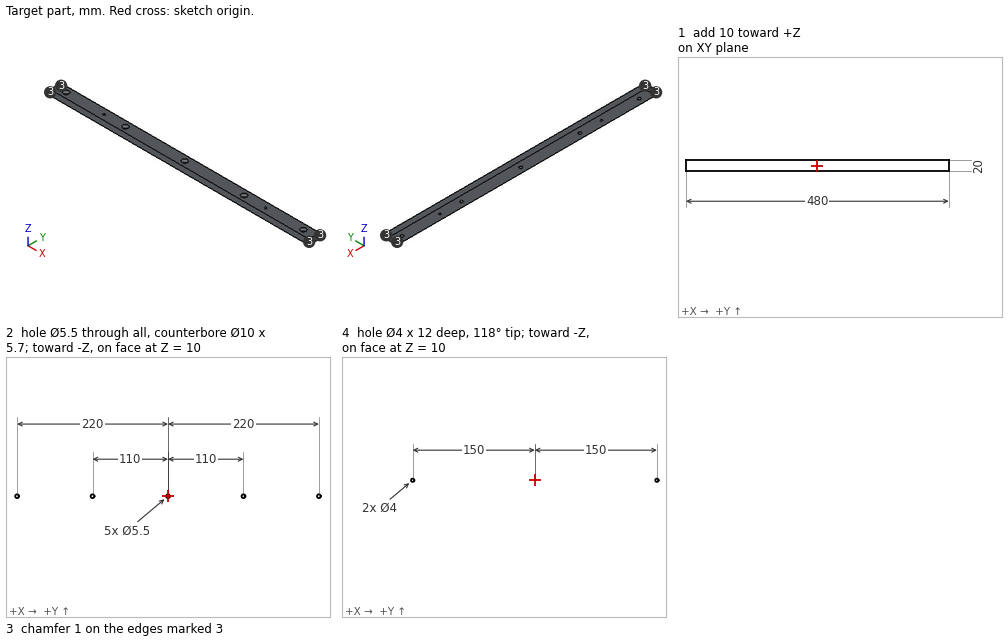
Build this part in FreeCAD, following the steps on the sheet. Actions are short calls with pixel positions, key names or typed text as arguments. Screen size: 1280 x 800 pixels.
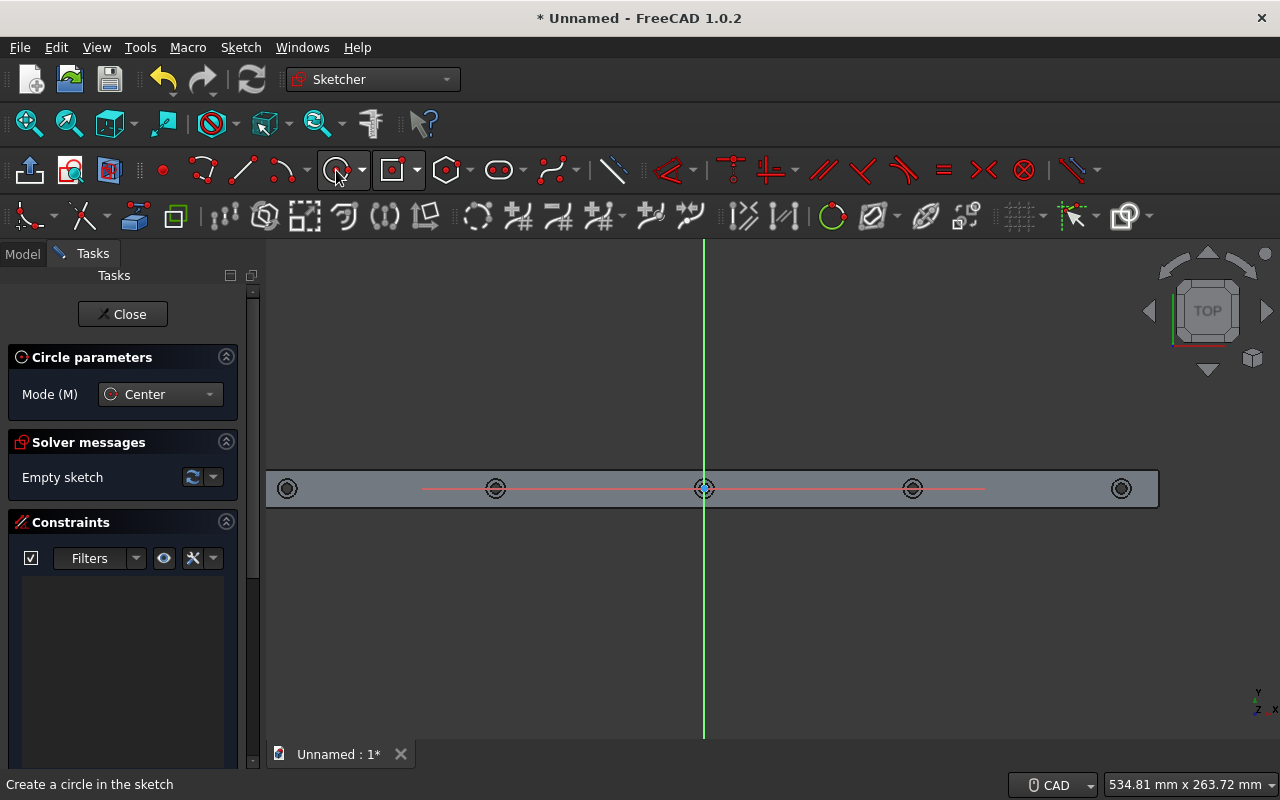
scroll(420, 489, up, 9)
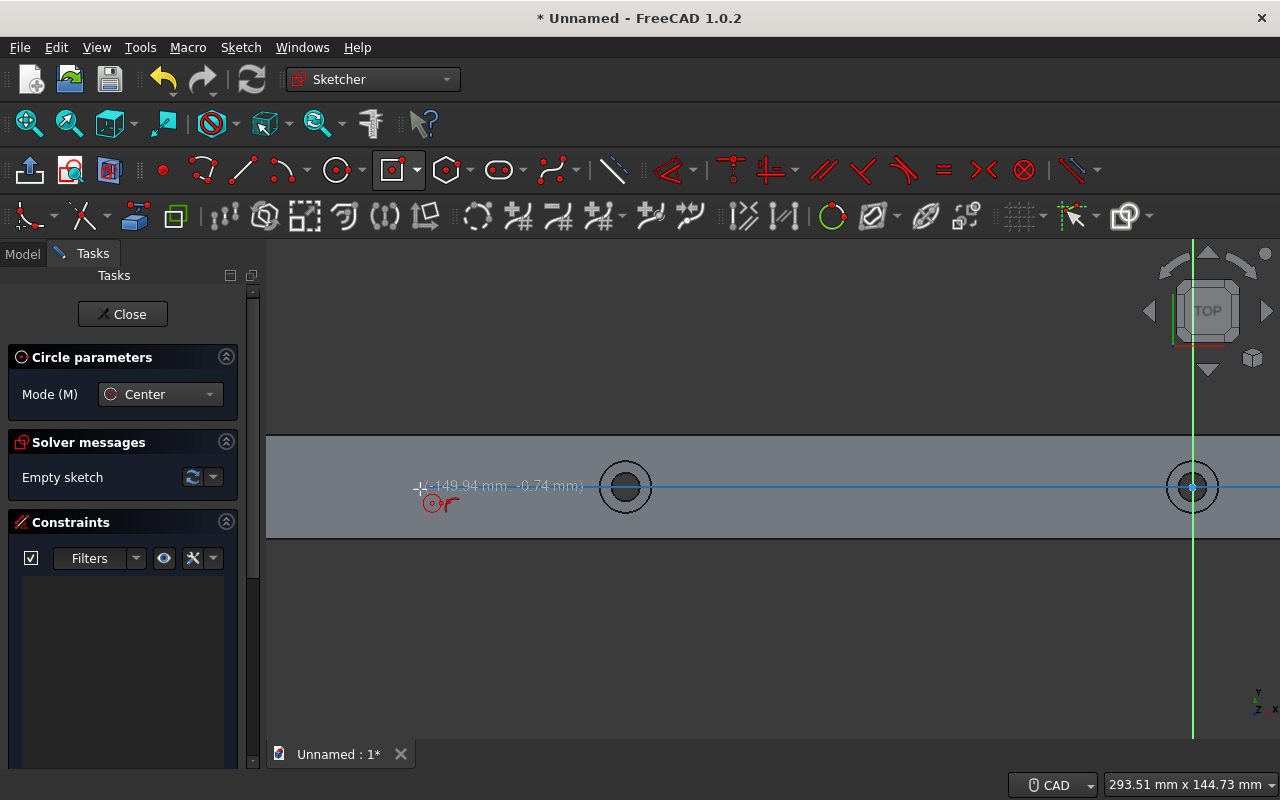
scroll(420, 490, down, 9)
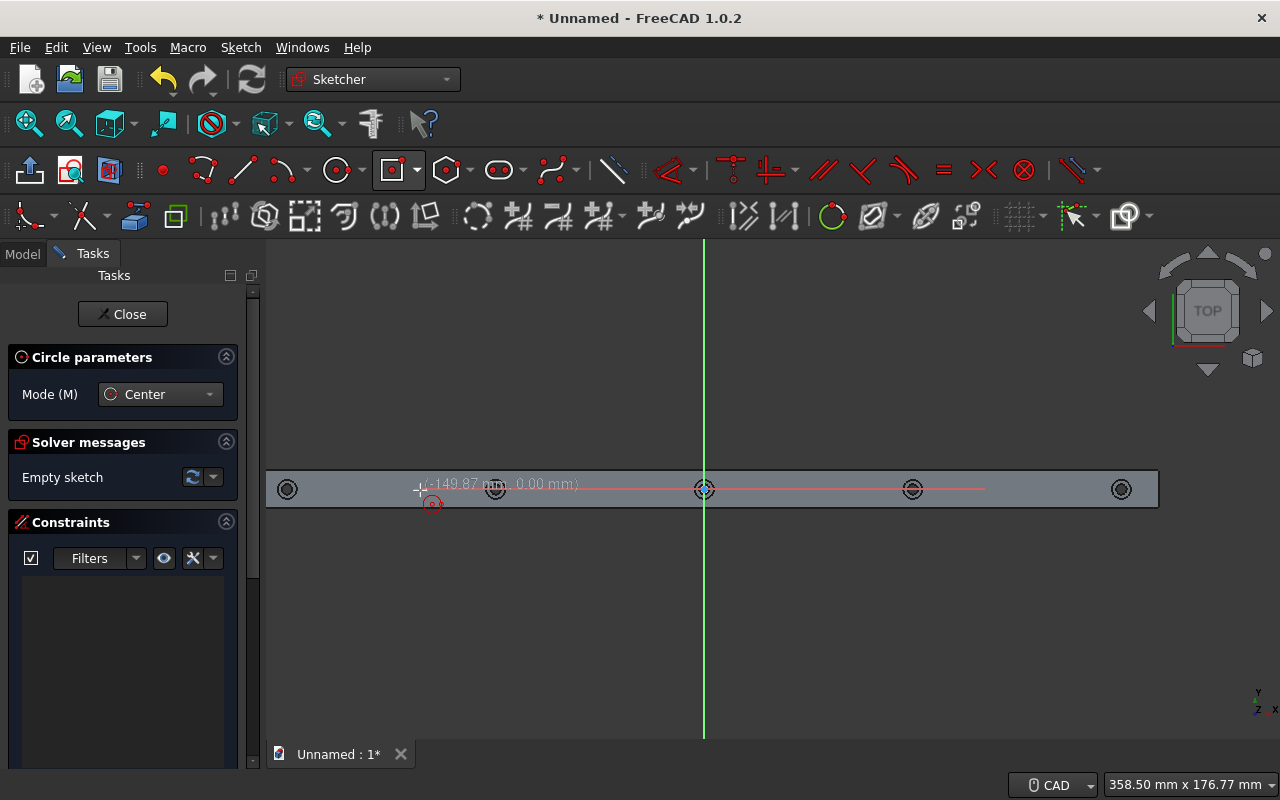
click(420, 489)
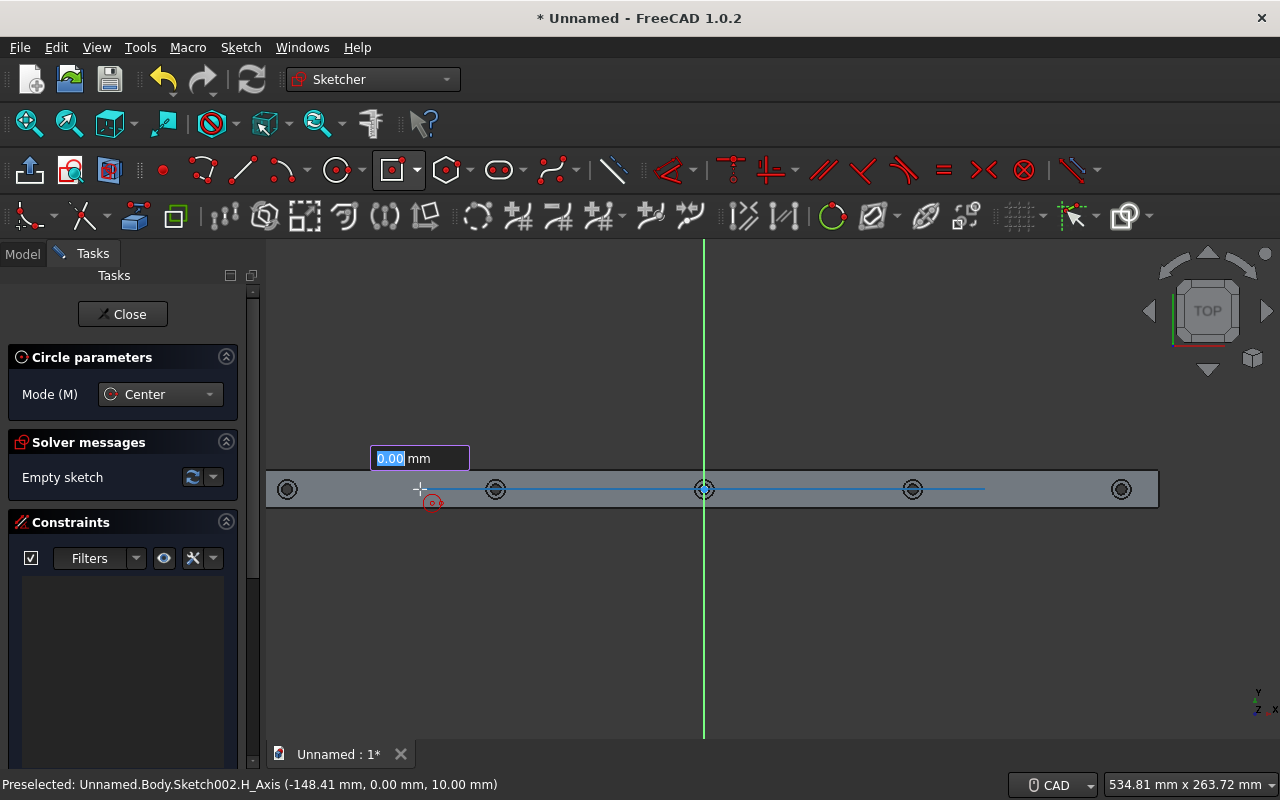
scroll(419, 493, up, 8)
move(416, 491)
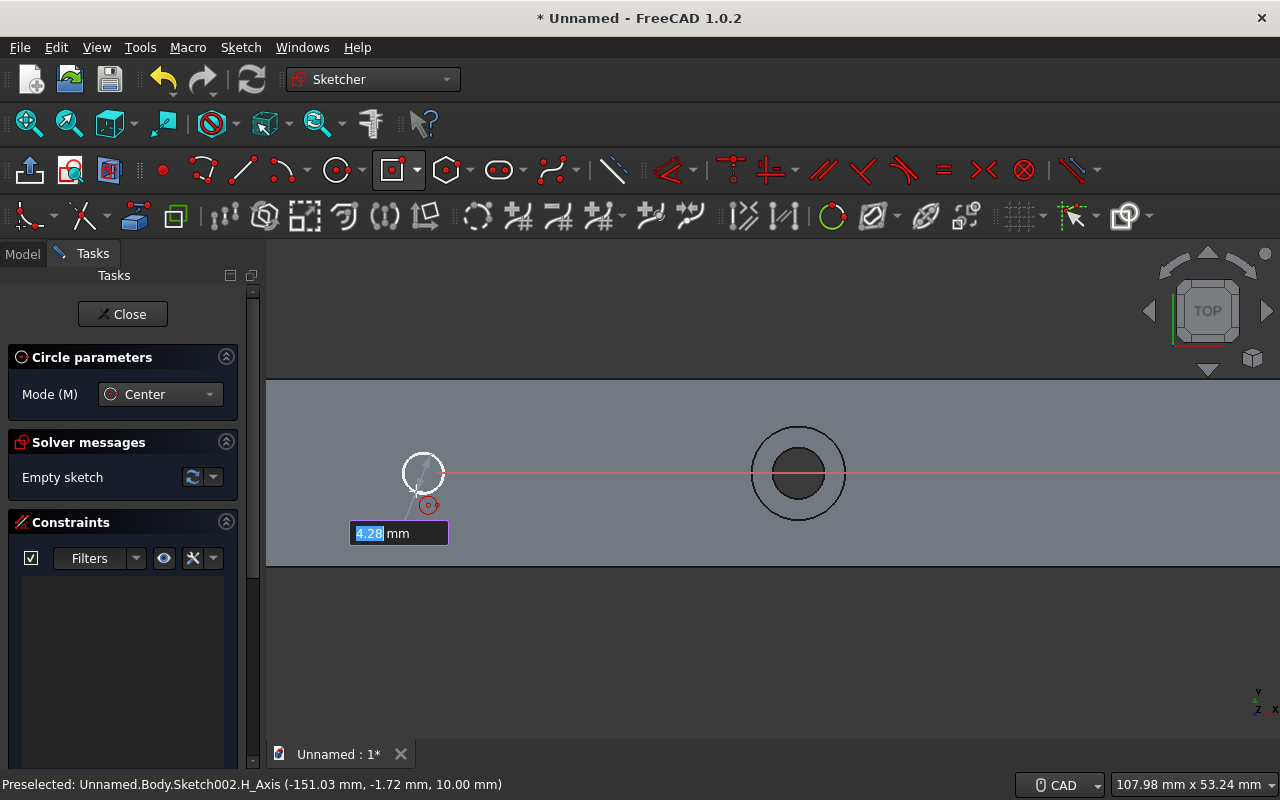
text(4)
key(Return)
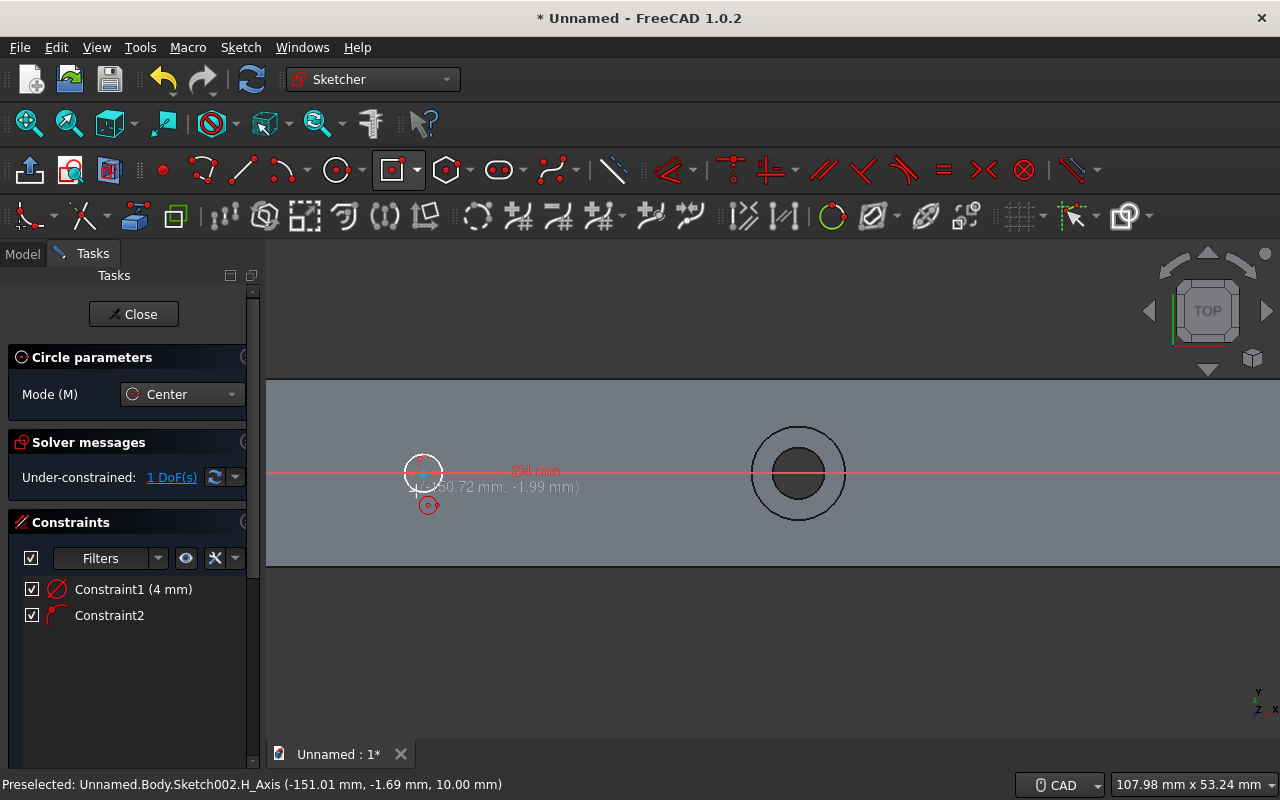
scroll(419, 493, down, 8)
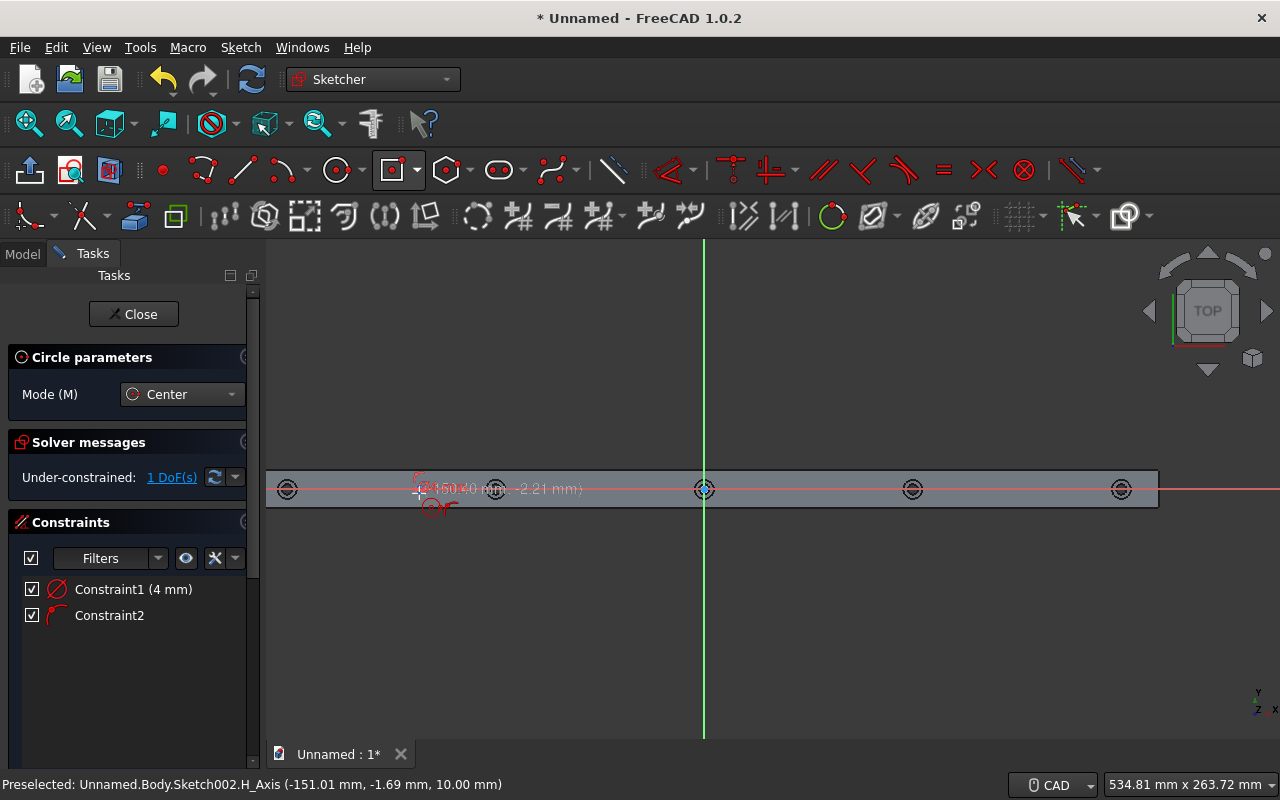
scroll(989, 489, up, 9)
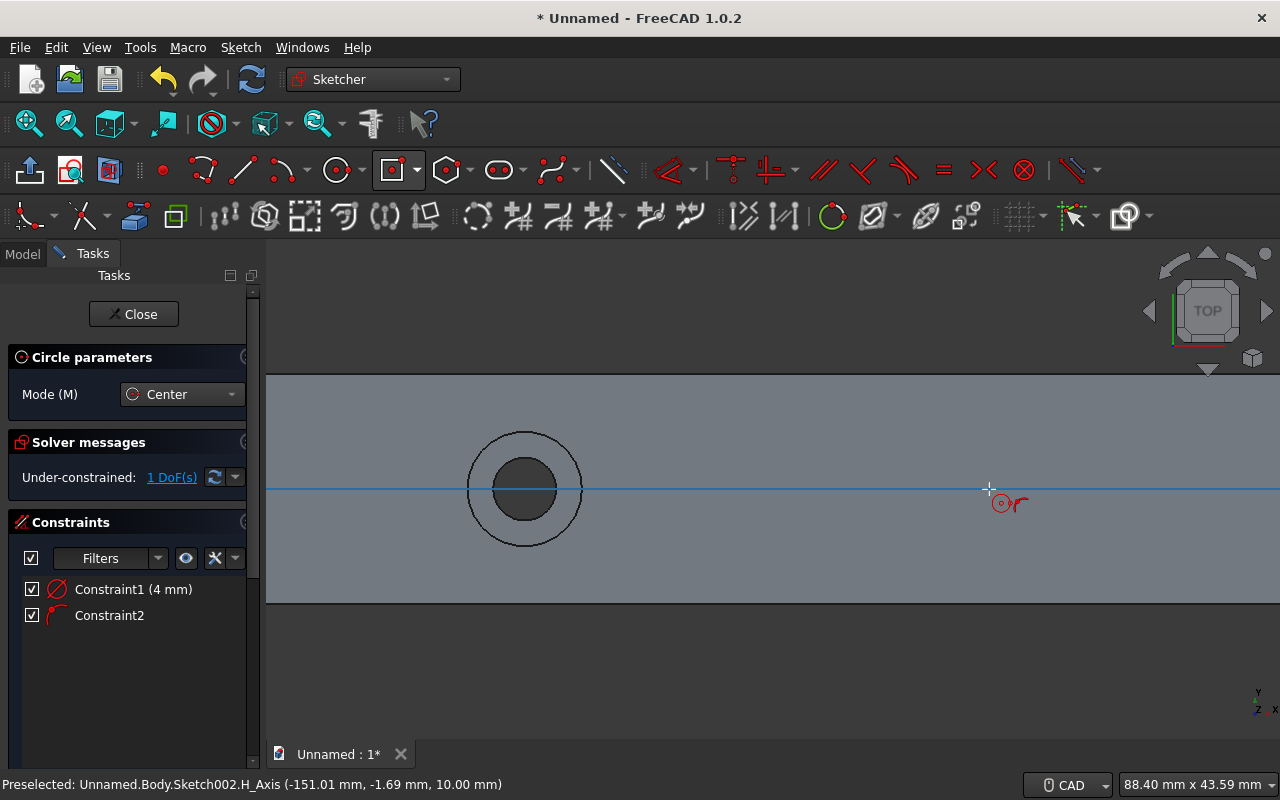
scroll(990, 489, down, 9)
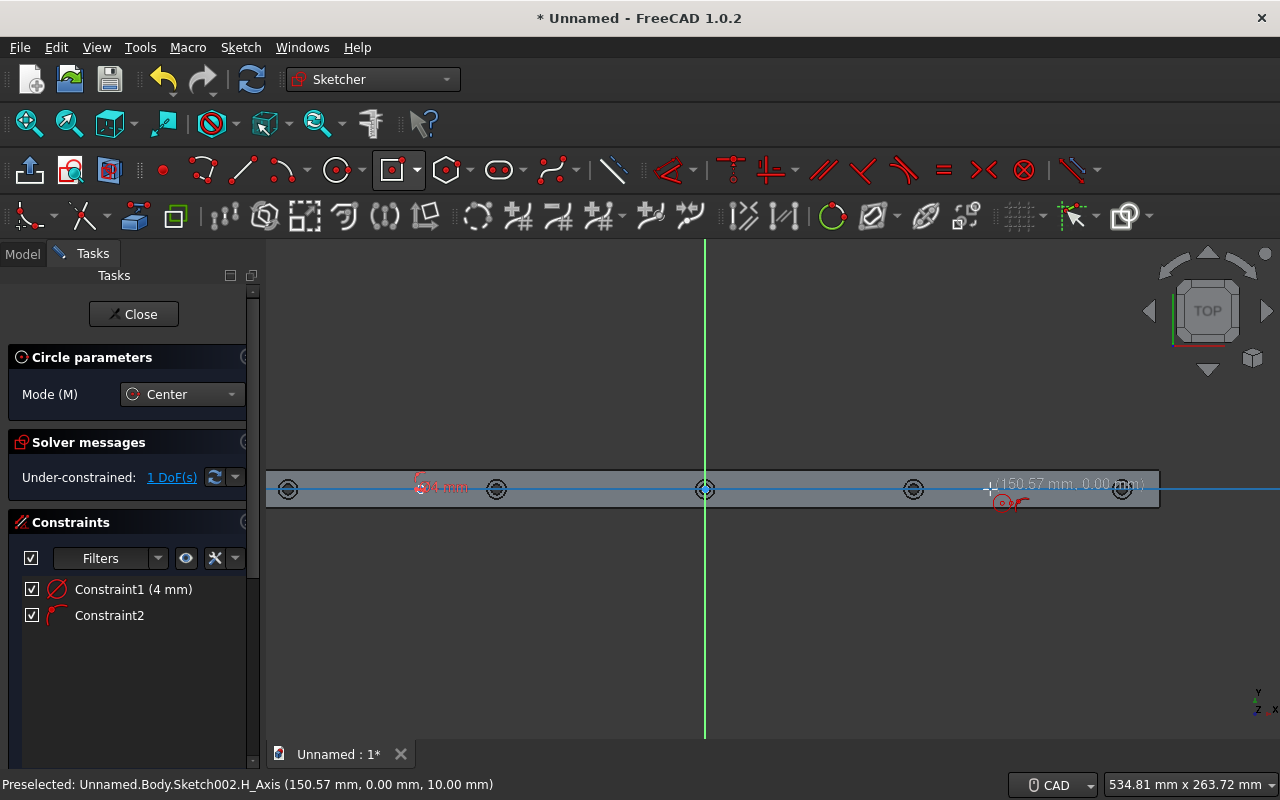
click(990, 489)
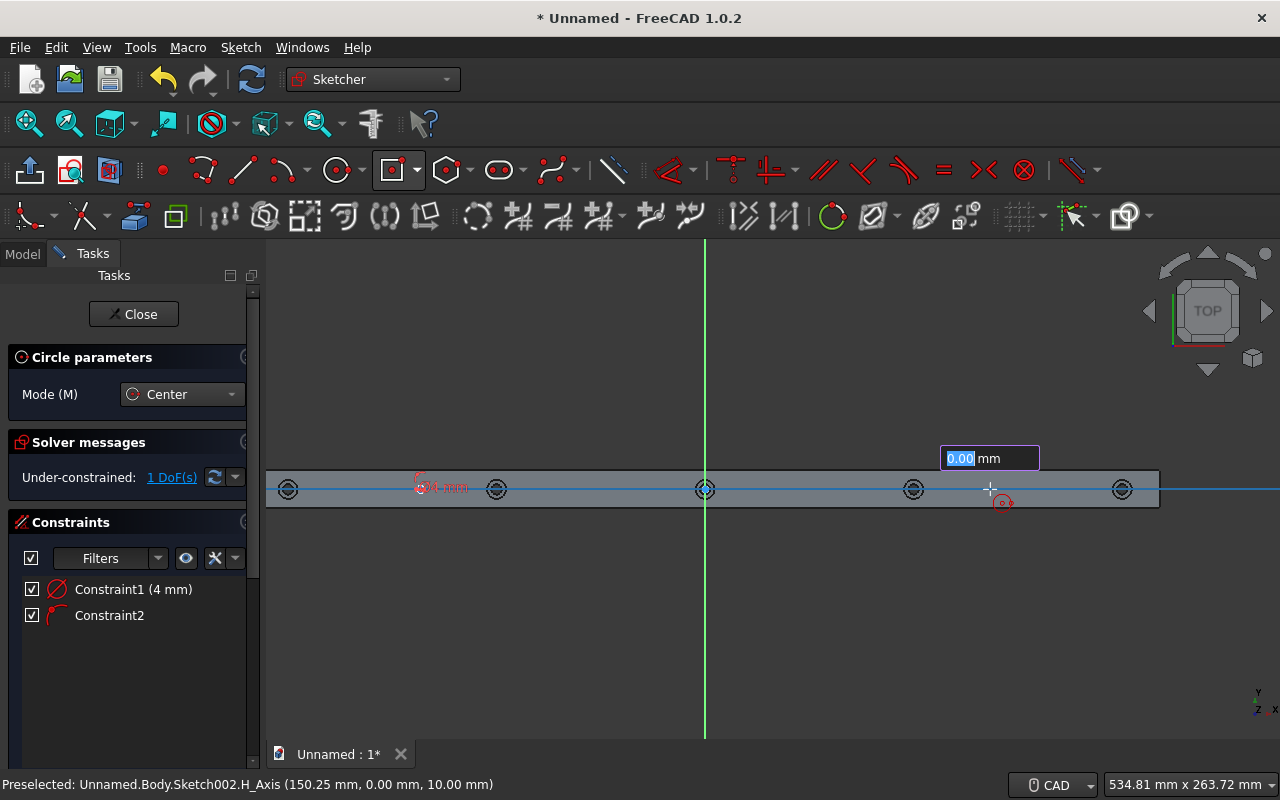
scroll(988, 493, up, 8)
move(986, 491)